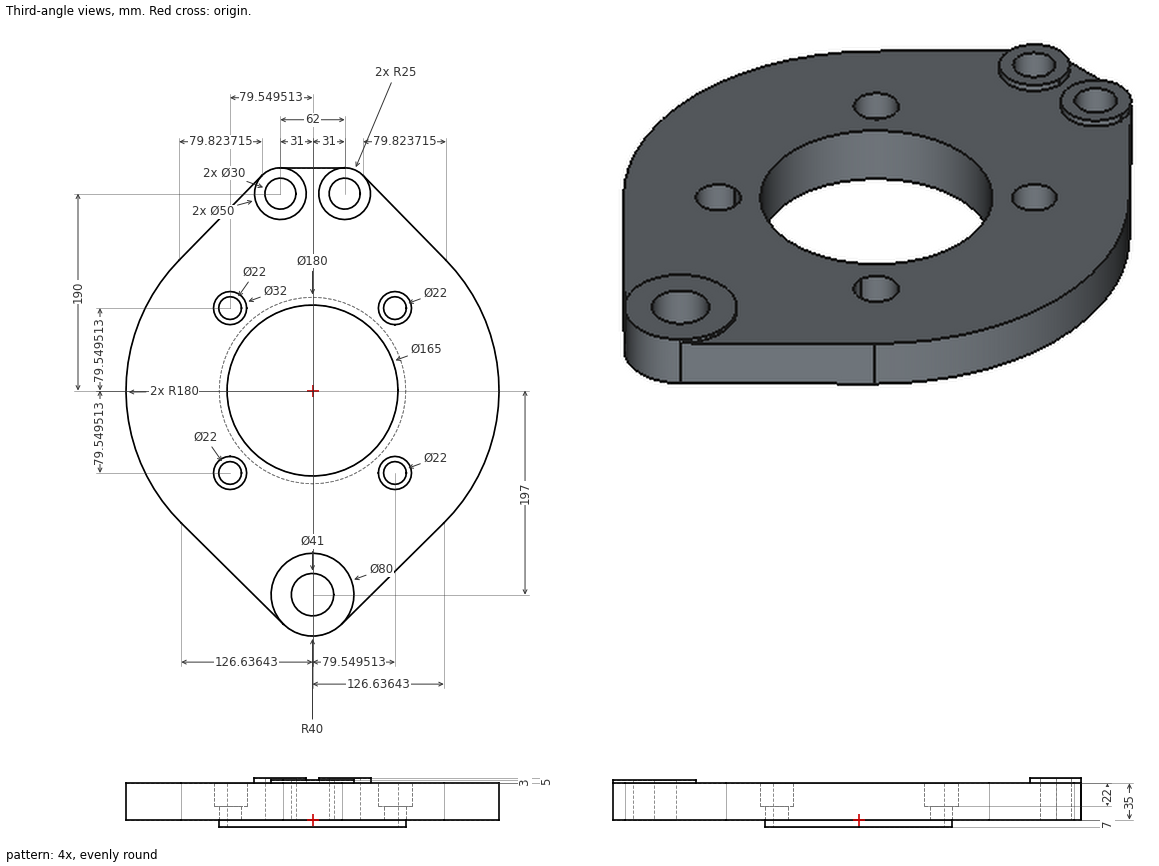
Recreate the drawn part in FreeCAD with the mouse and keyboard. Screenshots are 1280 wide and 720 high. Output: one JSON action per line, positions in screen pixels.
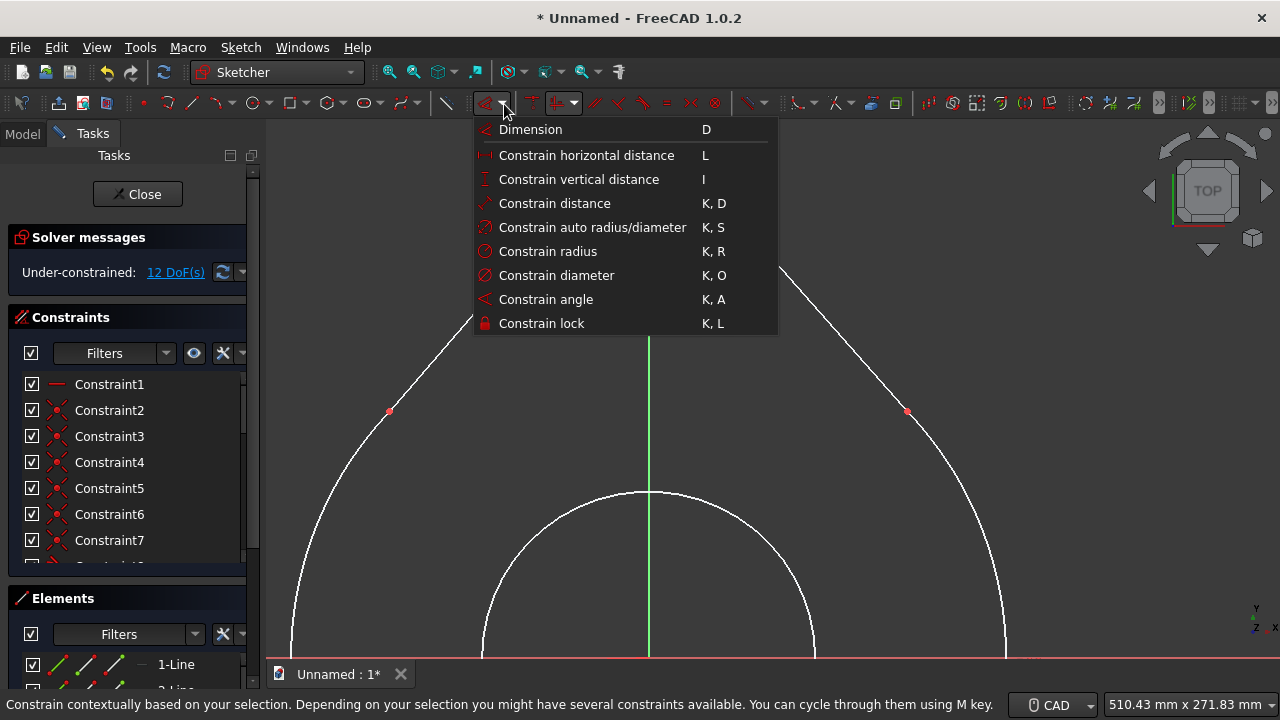
{"action": "left_click", "coordinate": [626, 251]}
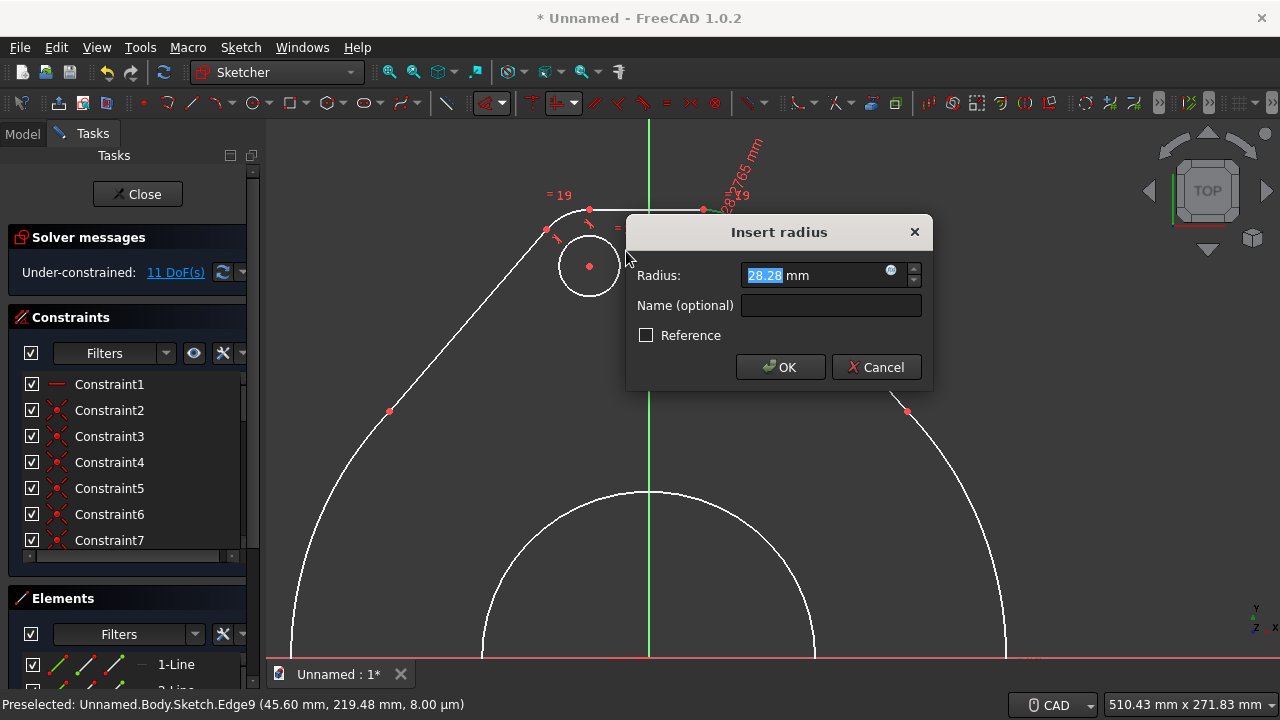
{"action": "type", "text": "25"}
{"action": "key", "text": "Return"}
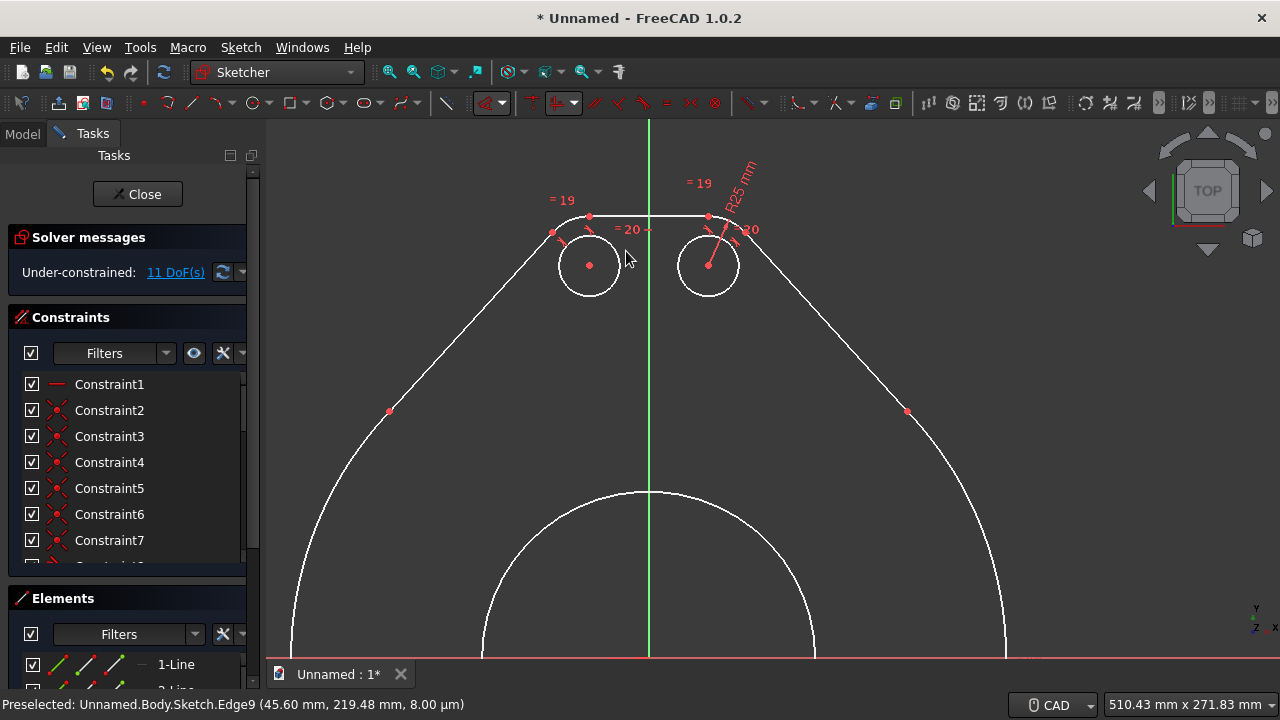
{"action": "scroll", "coordinate": [737, 220], "scroll_direction": "down", "scroll_amount": 5}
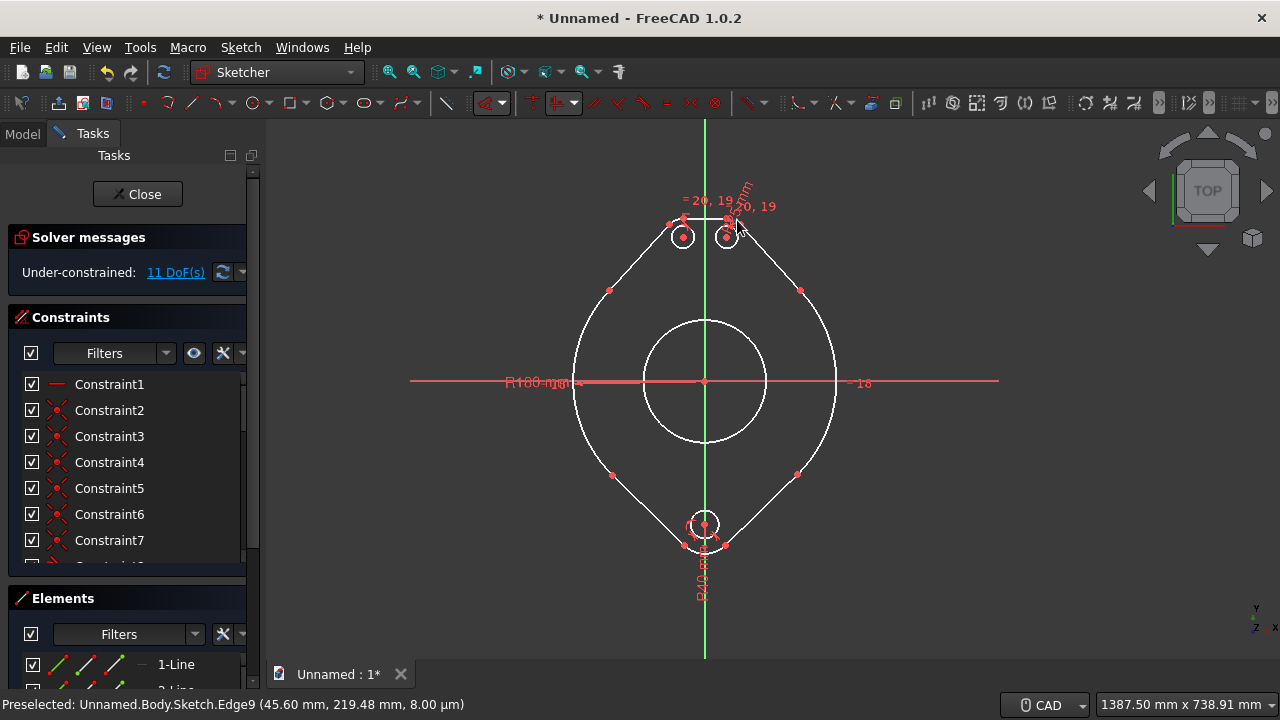
{"action": "scroll", "coordinate": [715, 515], "scroll_direction": "up", "scroll_amount": 2}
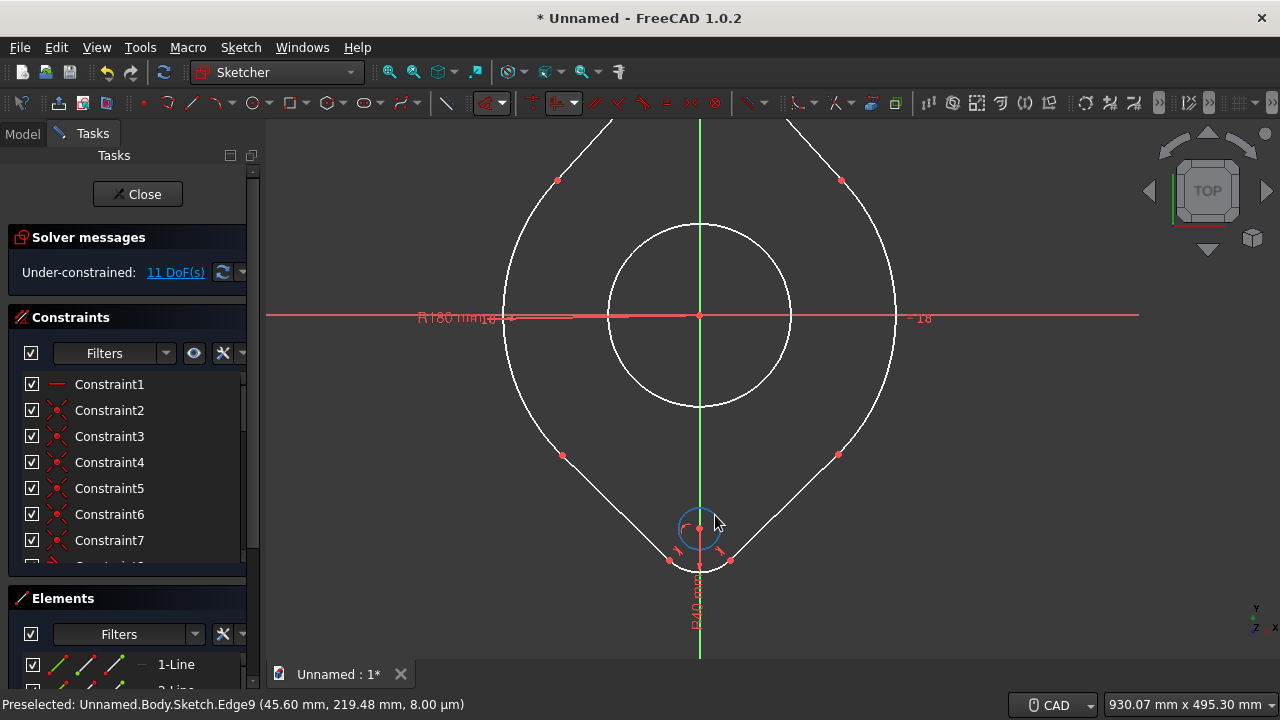
{"action": "left_click", "coordinate": [714, 514]}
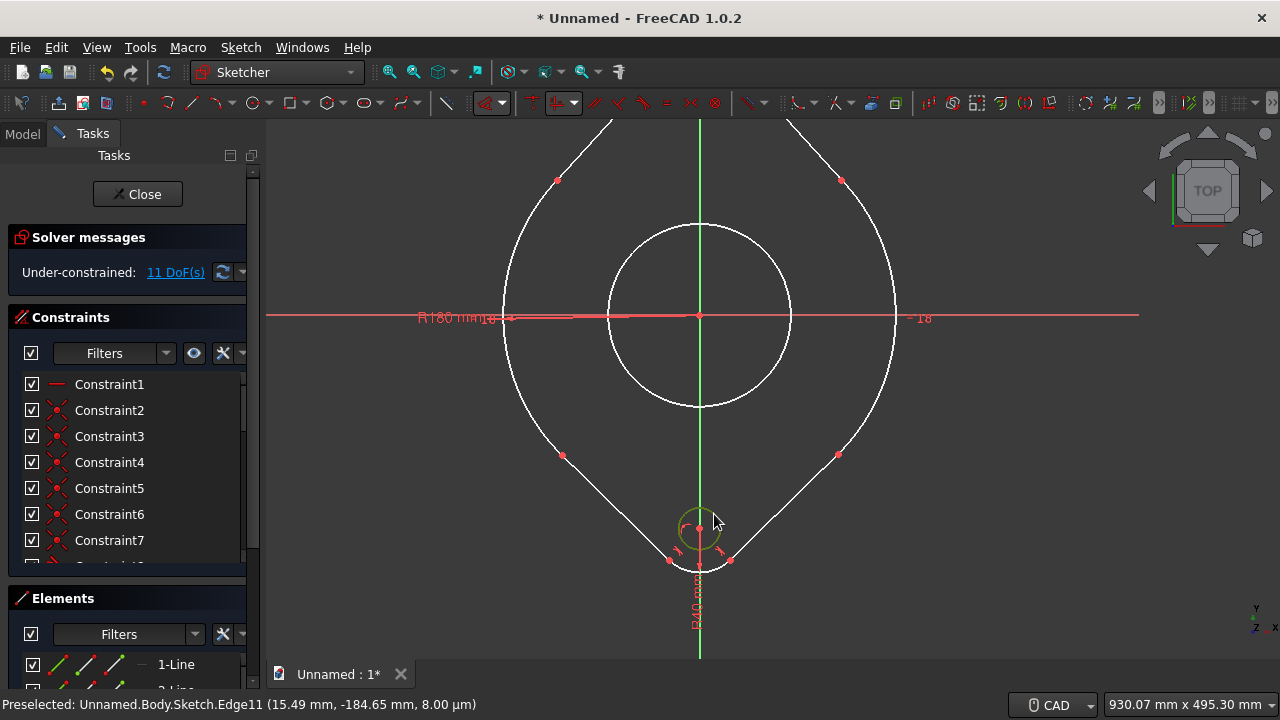
{"action": "key", "text": "k o"}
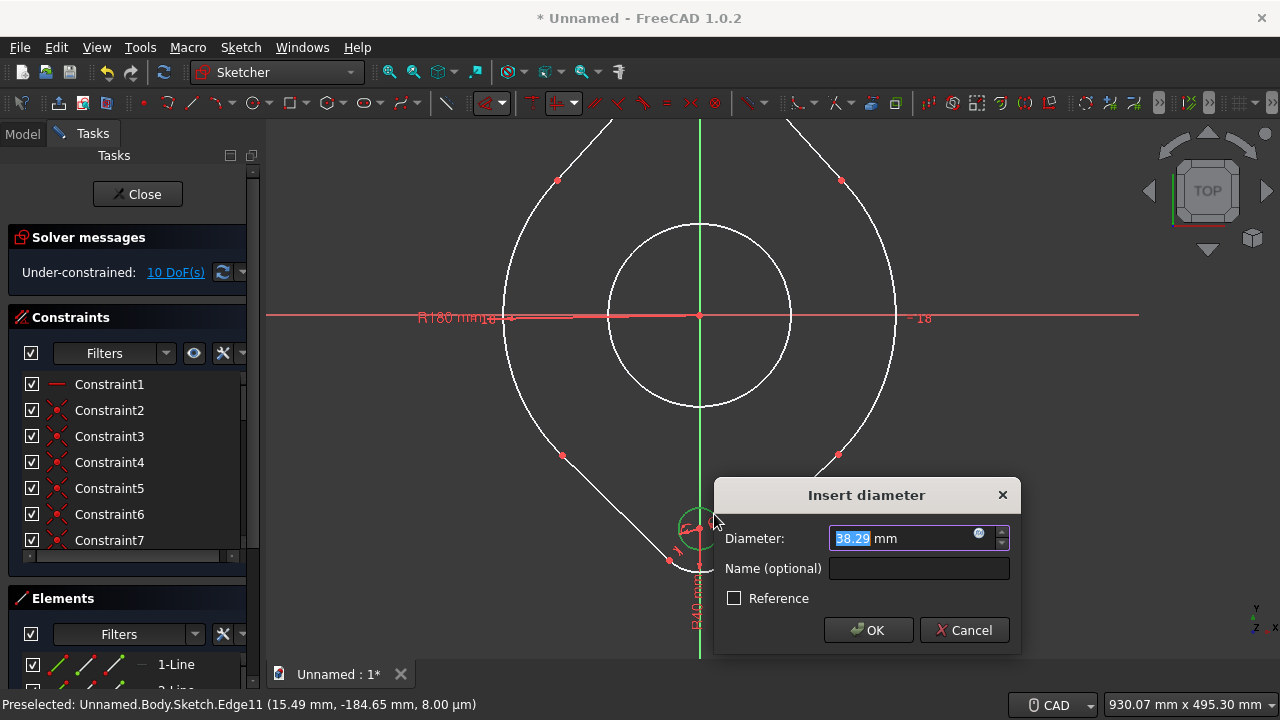
{"action": "type", "text": "41"}
{"action": "key", "text": "Return"}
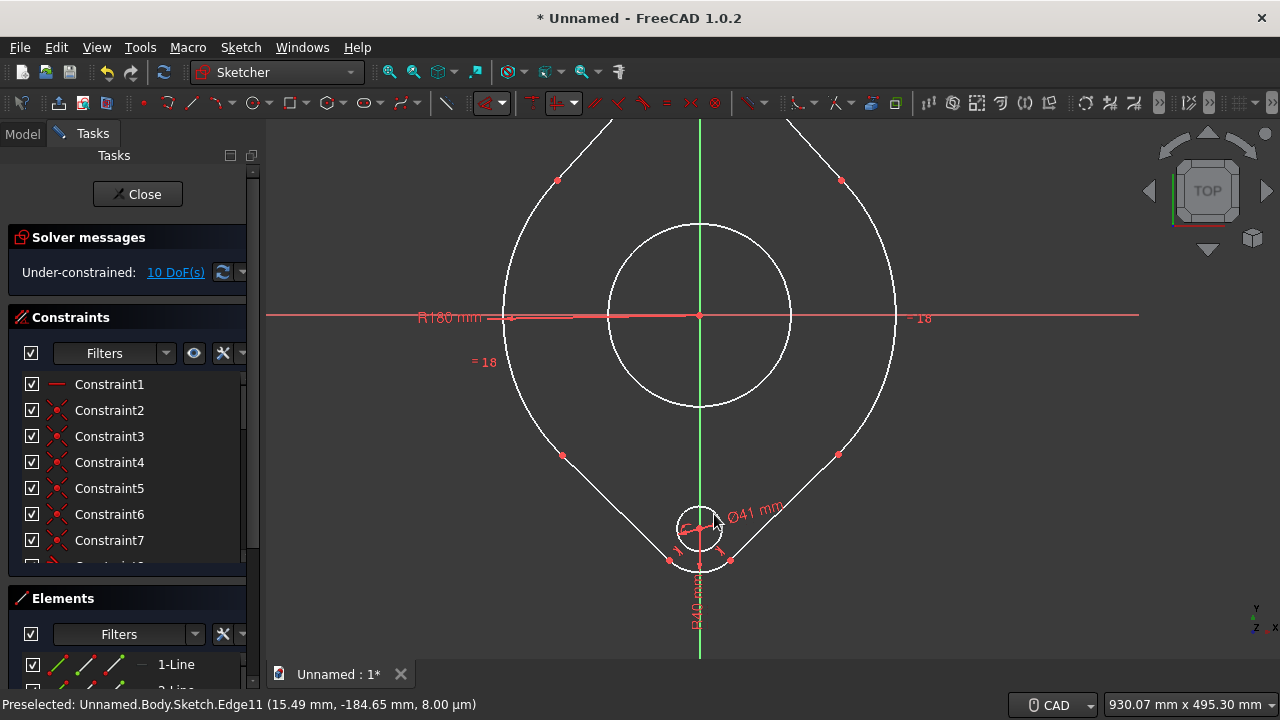
{"action": "scroll", "coordinate": [715, 515], "scroll_direction": "down", "scroll_amount": 2}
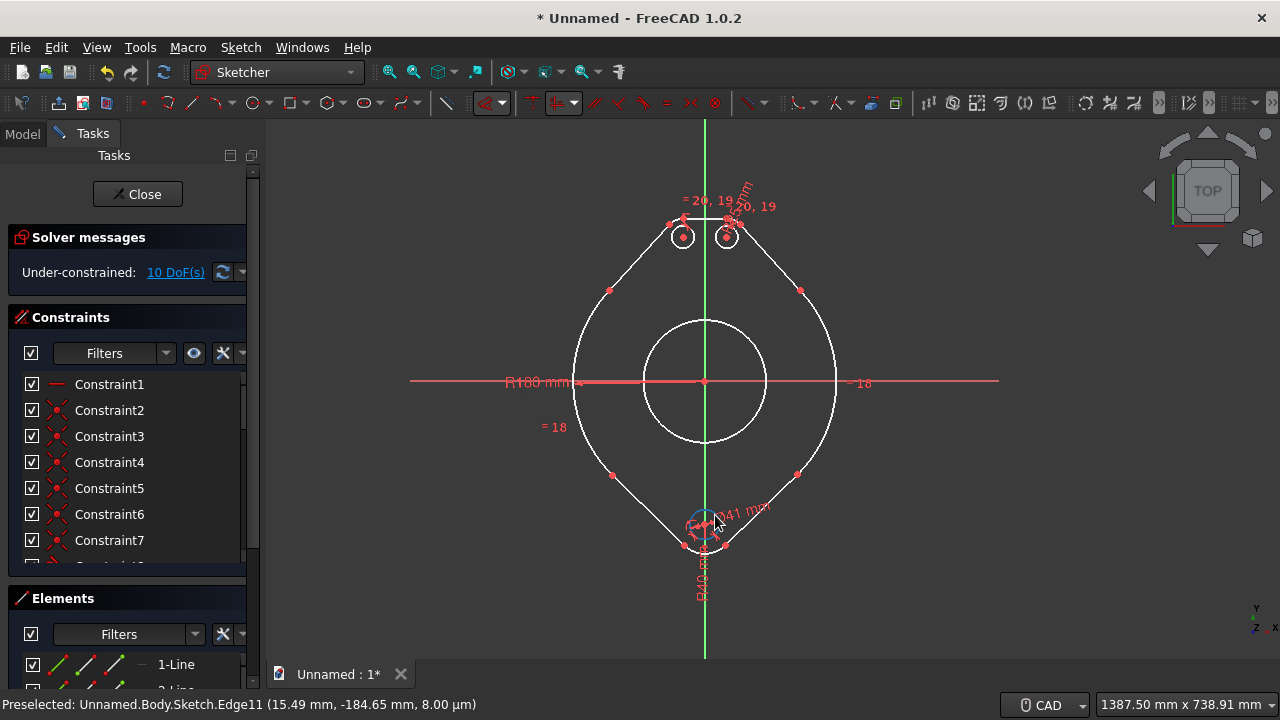
{"action": "scroll", "coordinate": [691, 229], "scroll_direction": "up", "scroll_amount": 3}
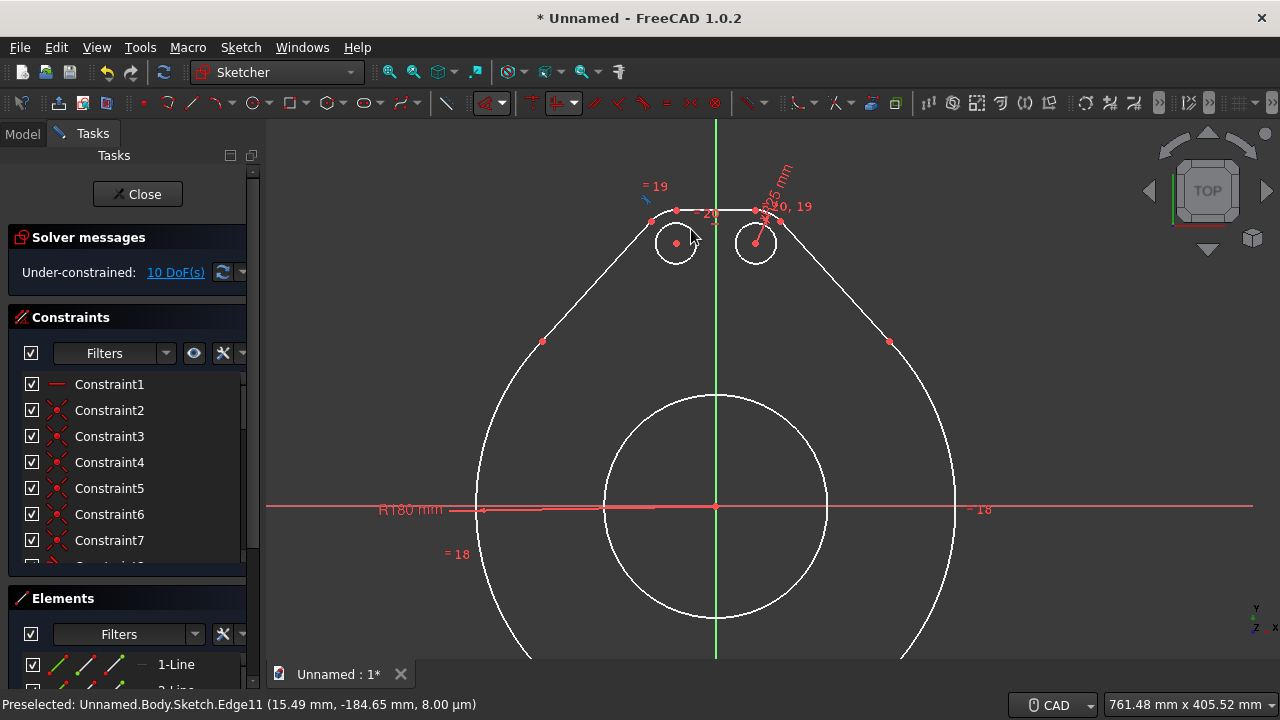
{"action": "left_click", "coordinate": [690, 229]}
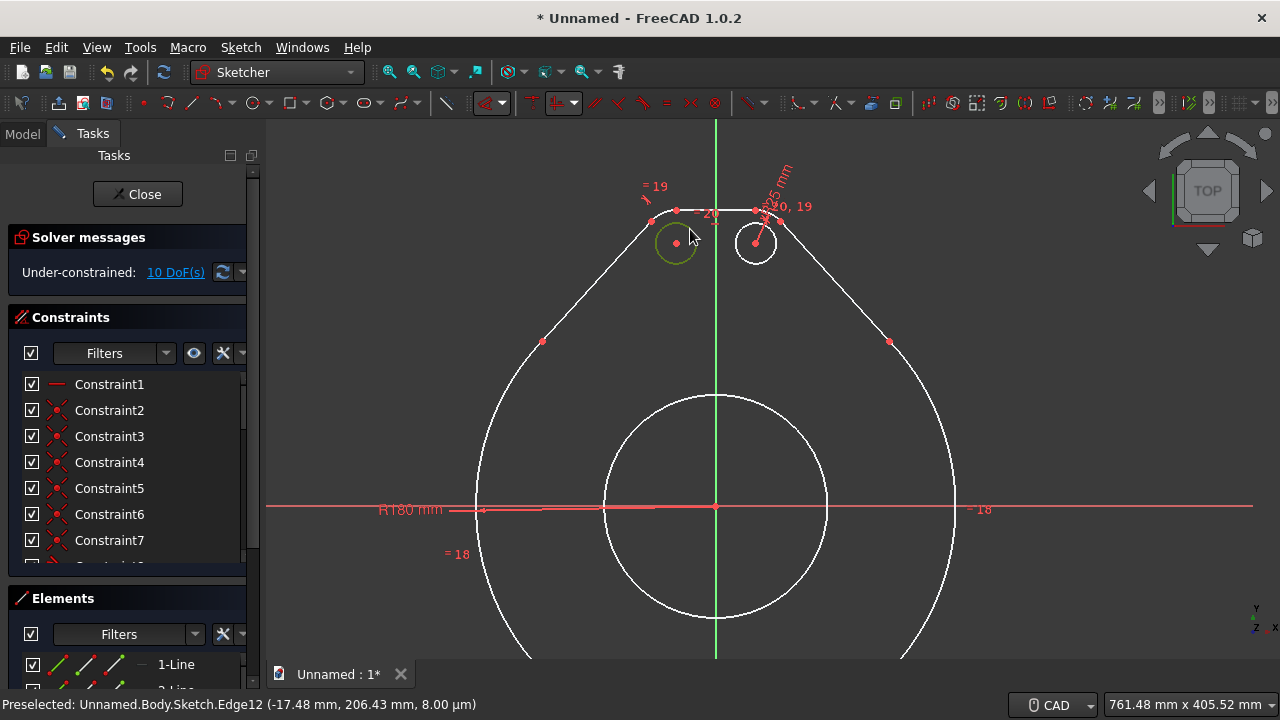
{"action": "key", "text": "k o"}